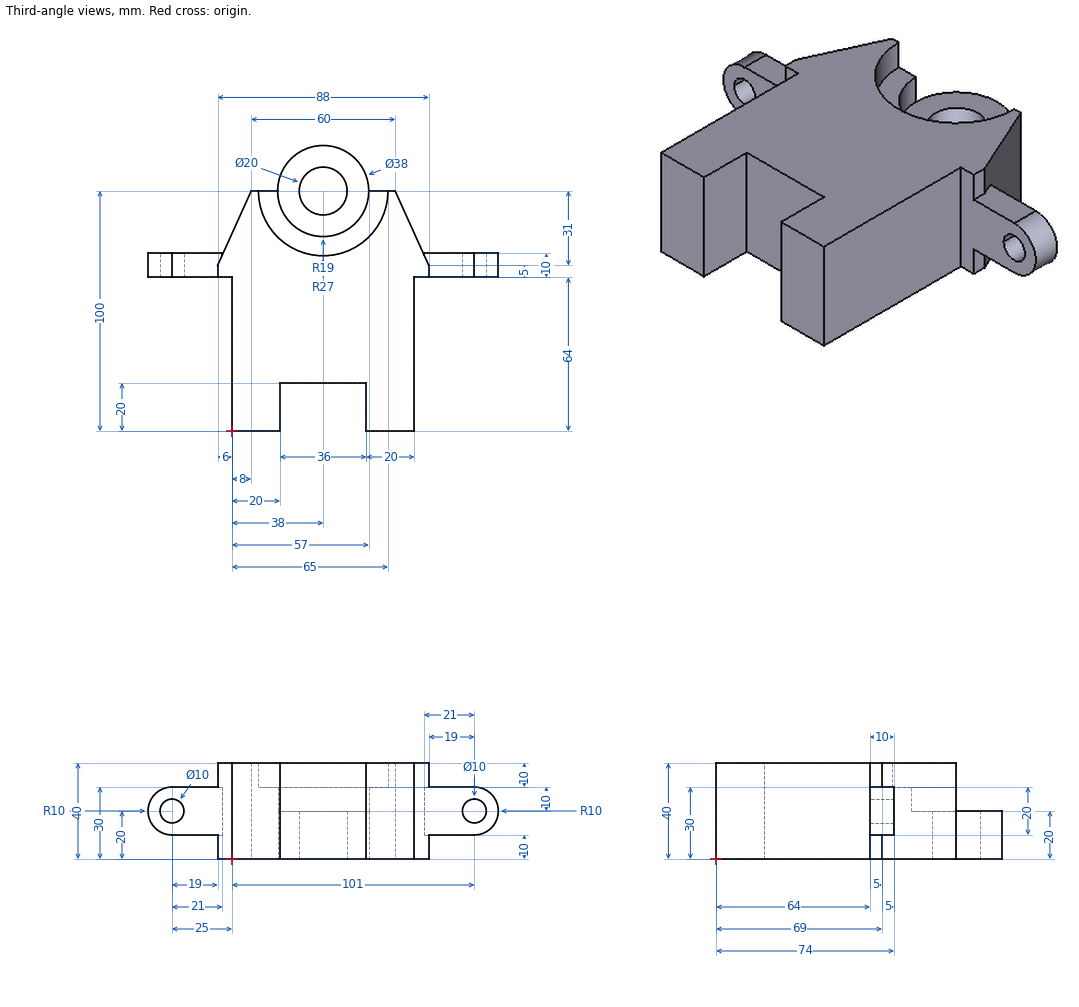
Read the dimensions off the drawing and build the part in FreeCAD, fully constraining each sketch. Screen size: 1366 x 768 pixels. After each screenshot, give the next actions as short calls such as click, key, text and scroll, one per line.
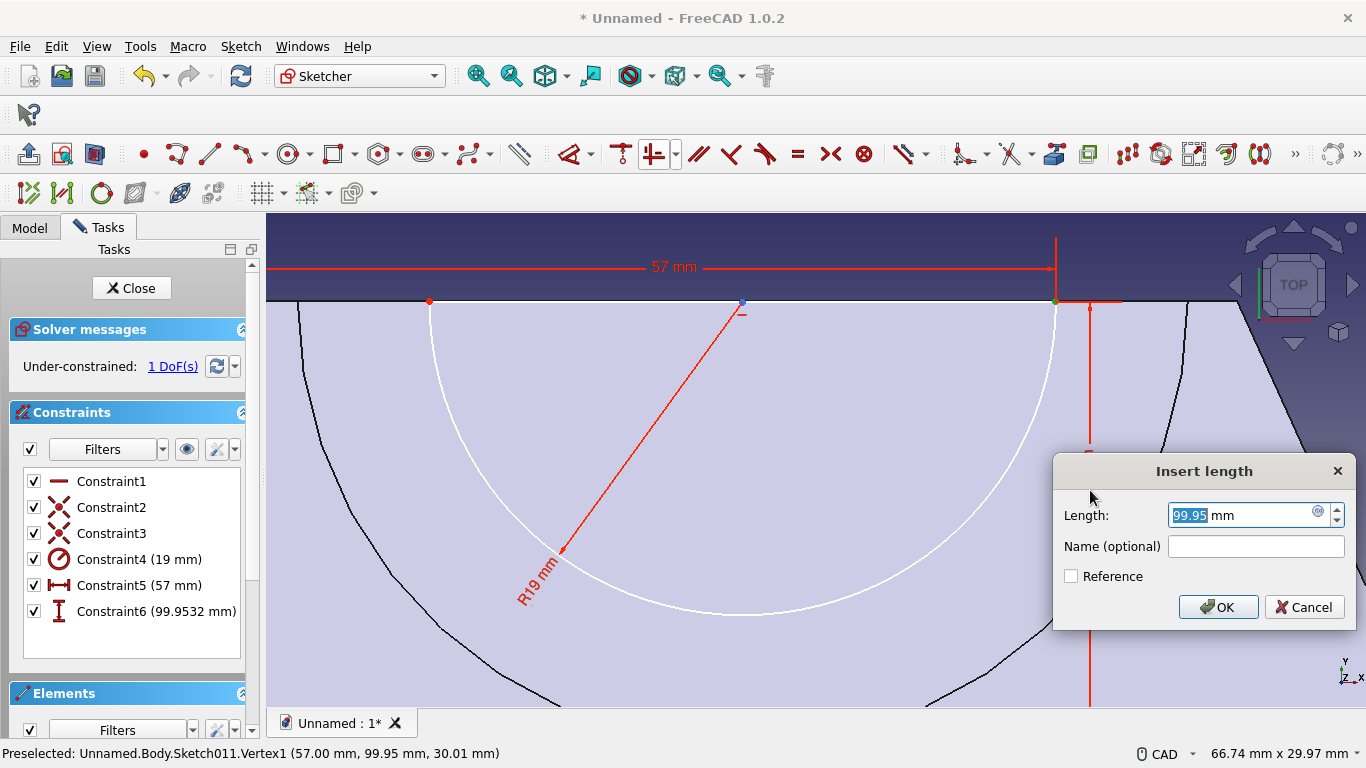
text(100)
key(Return)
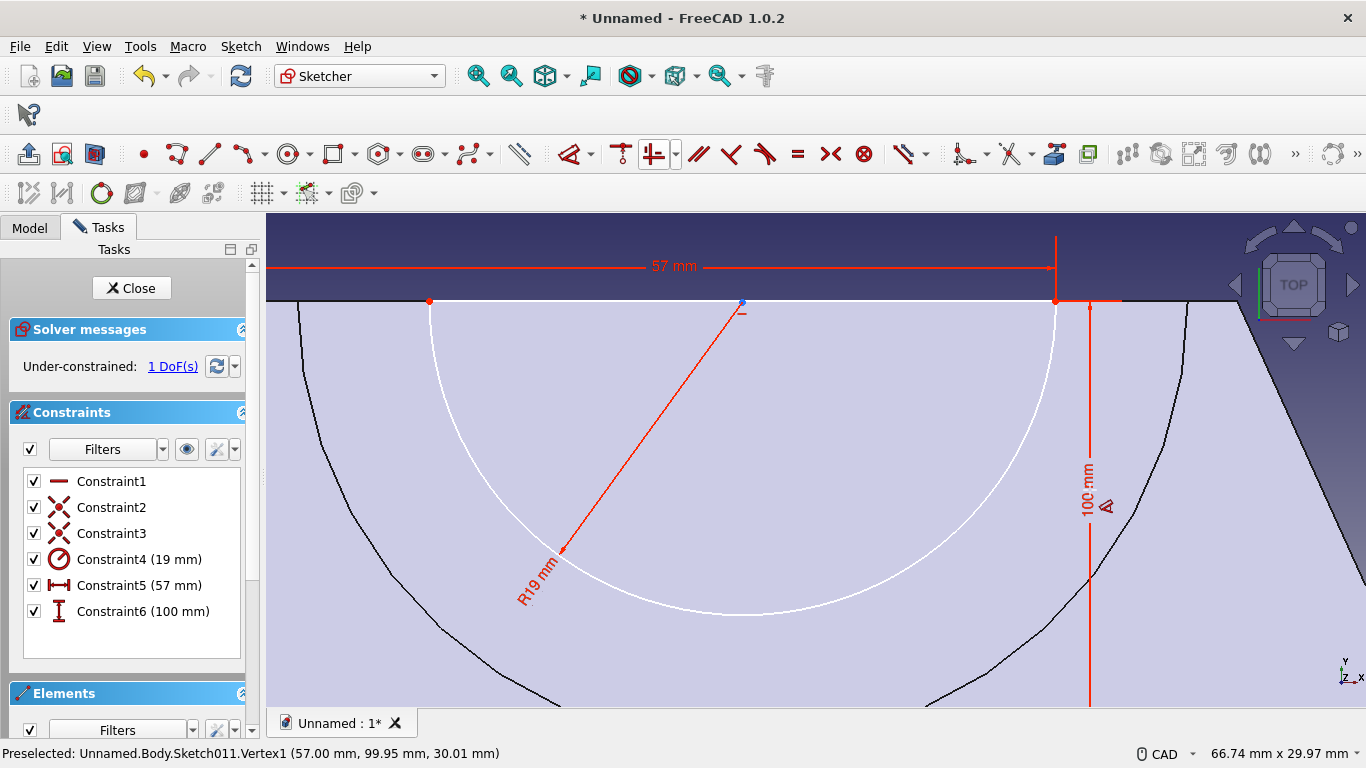
click(743, 302)
click(777, 491)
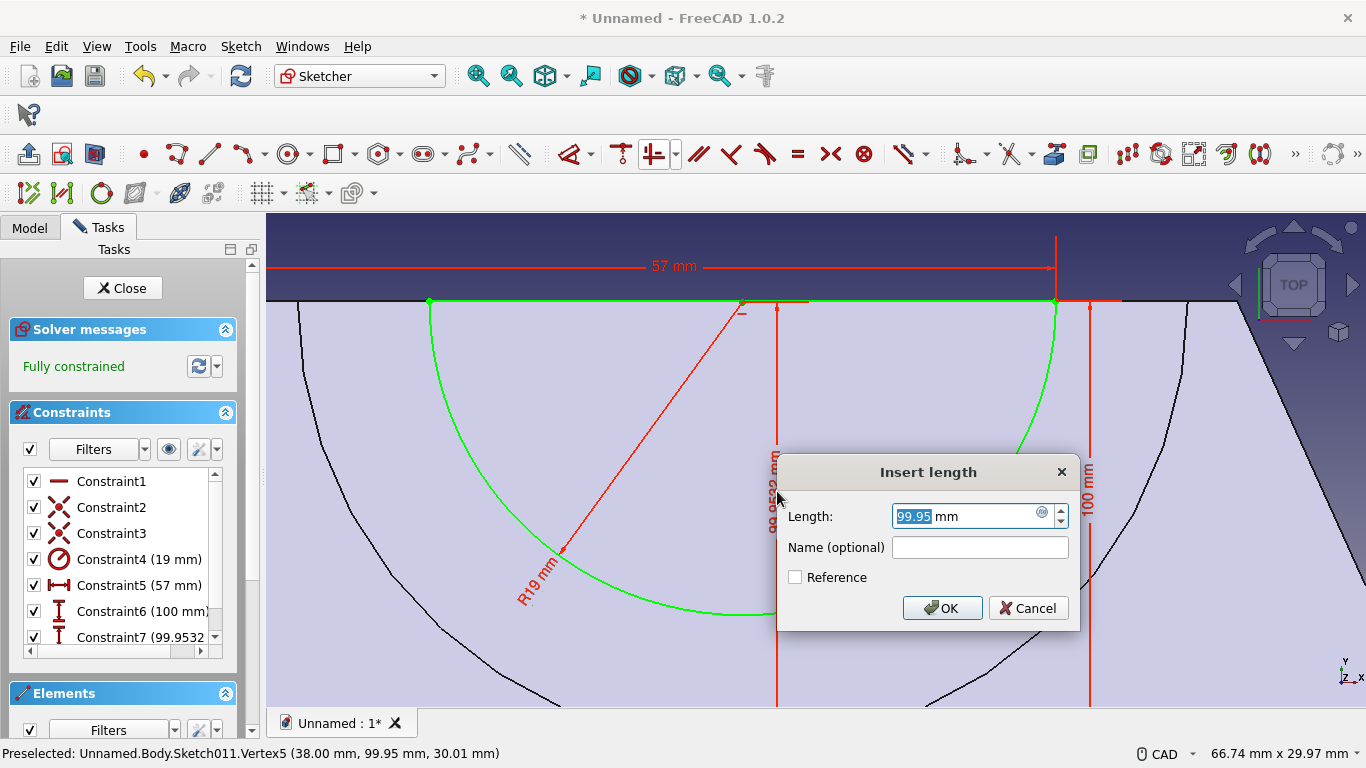
text(100)
key(Return)
key(Escape)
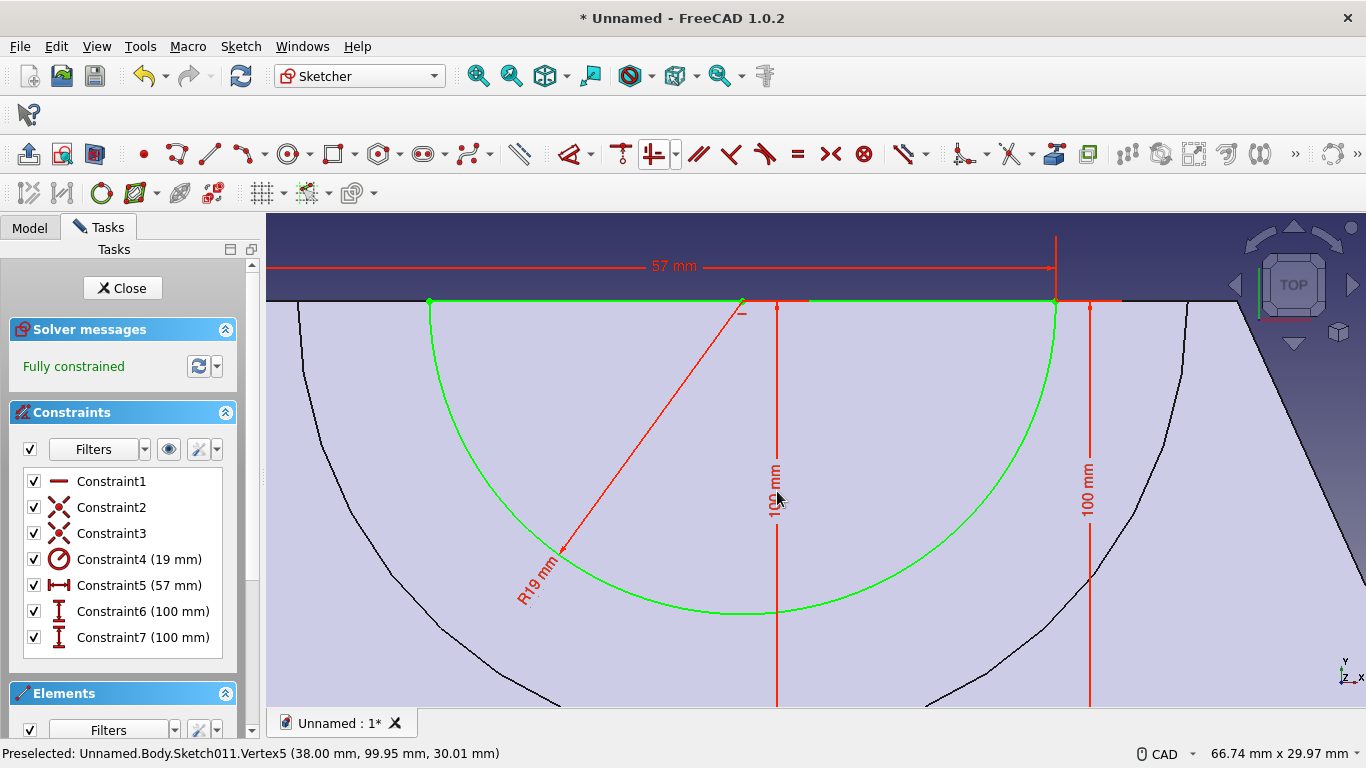
click(123, 288)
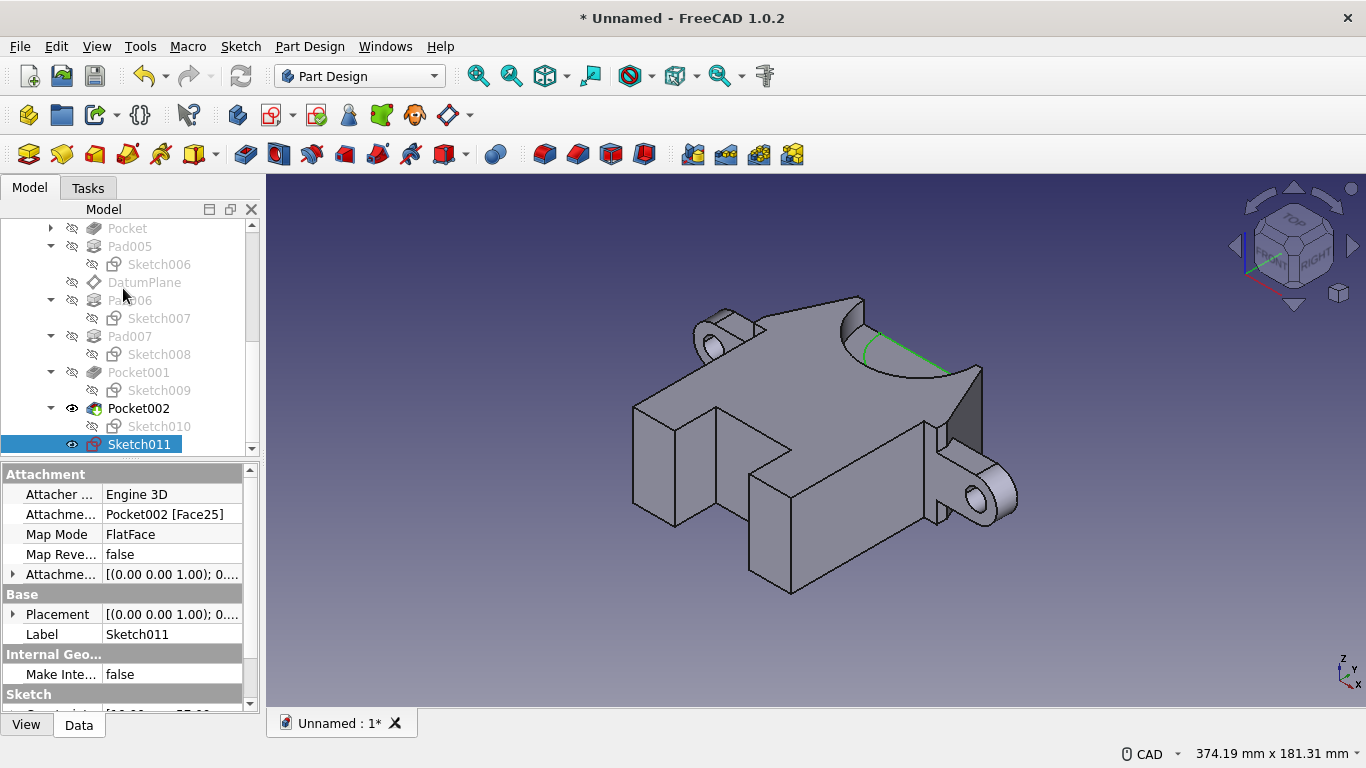
click(246, 154)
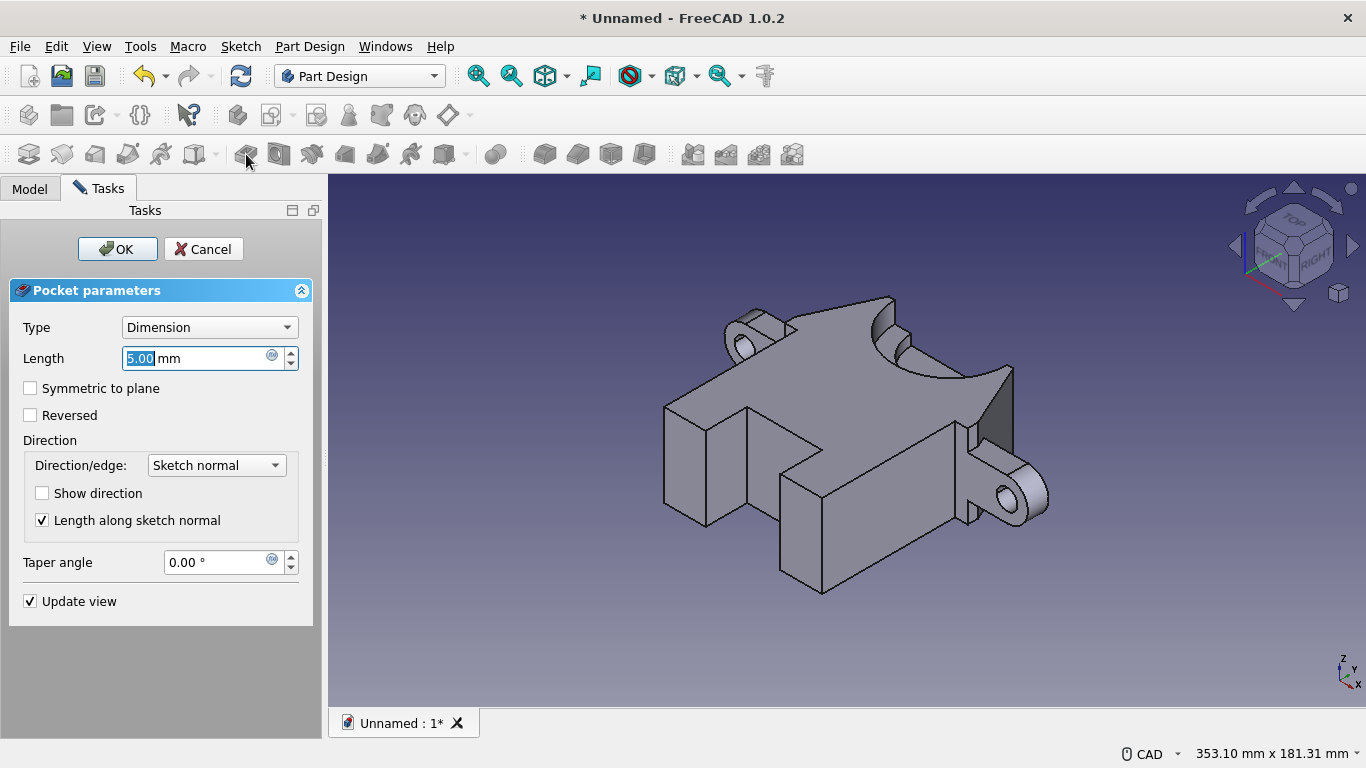
text(30)
key(Tab)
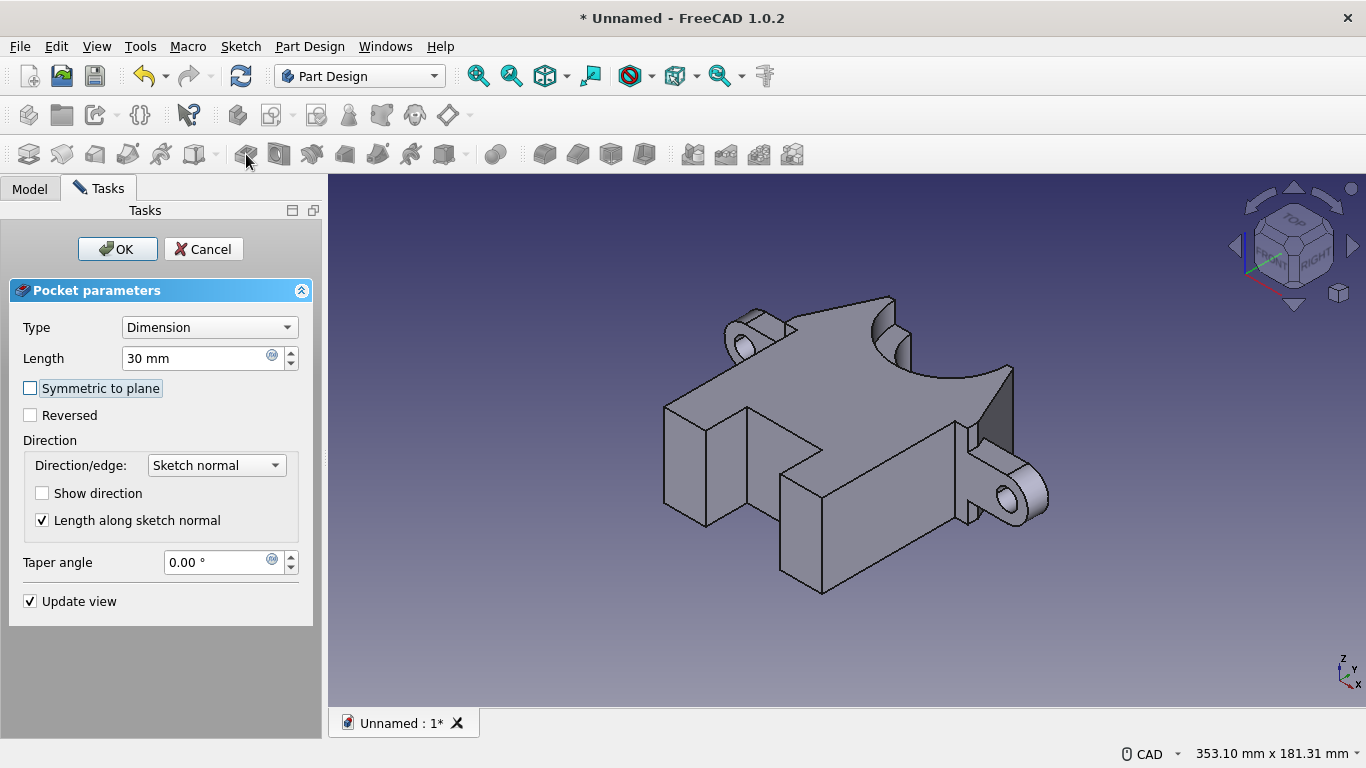
click(118, 249)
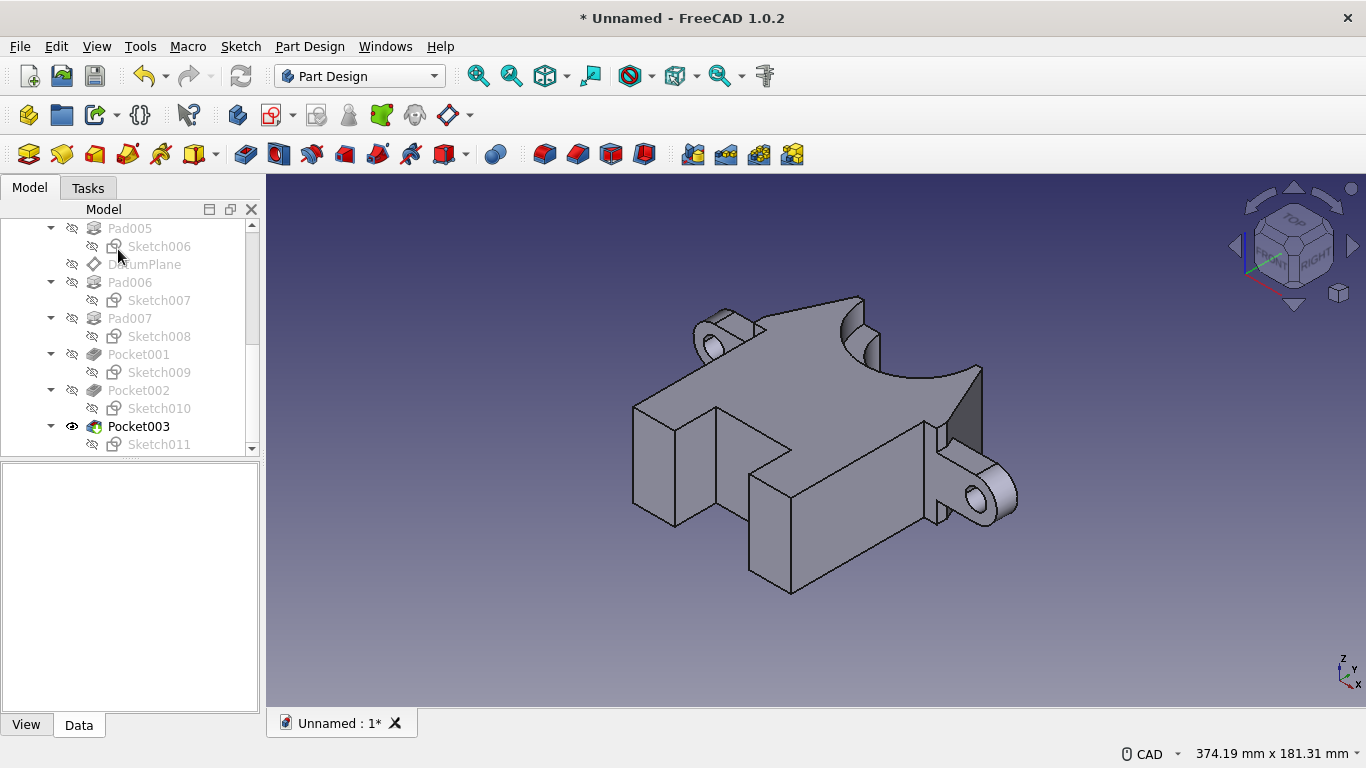
click(860, 335)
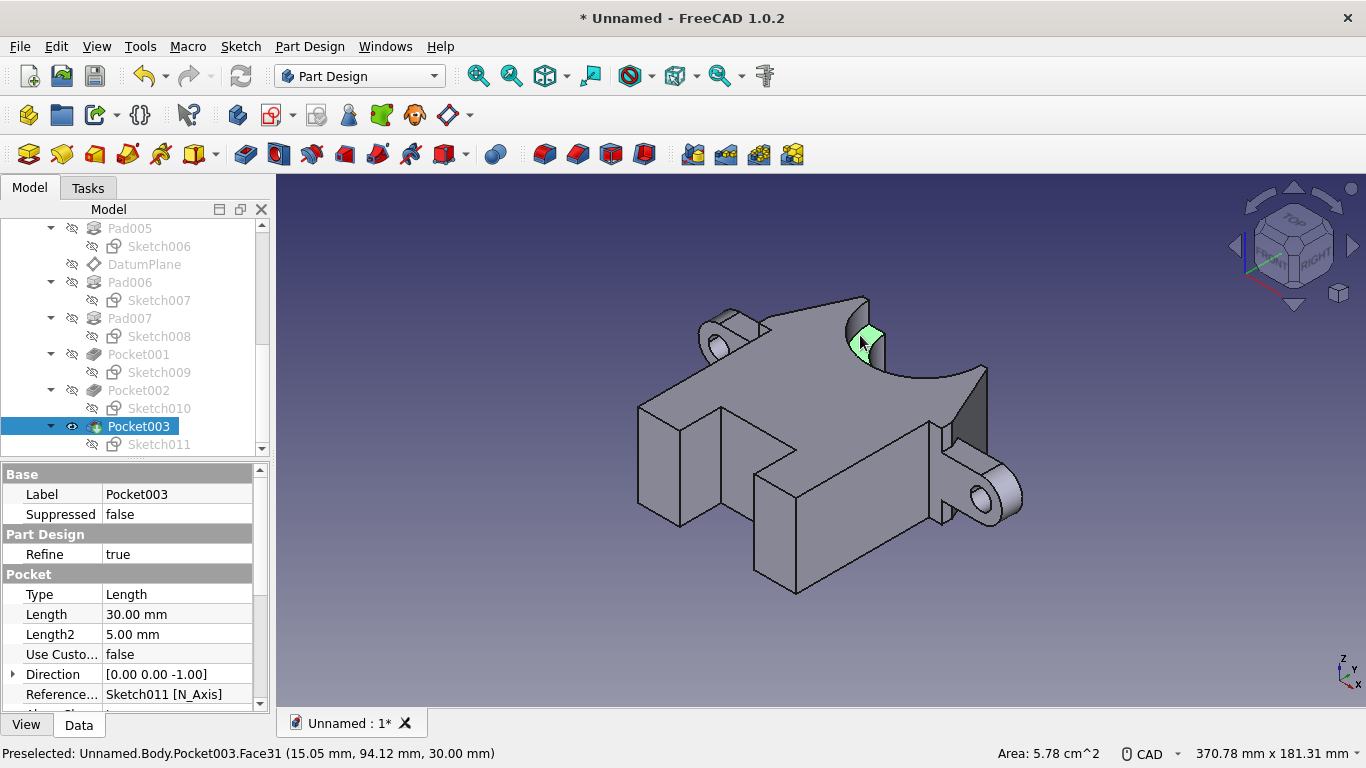
click(270, 116)